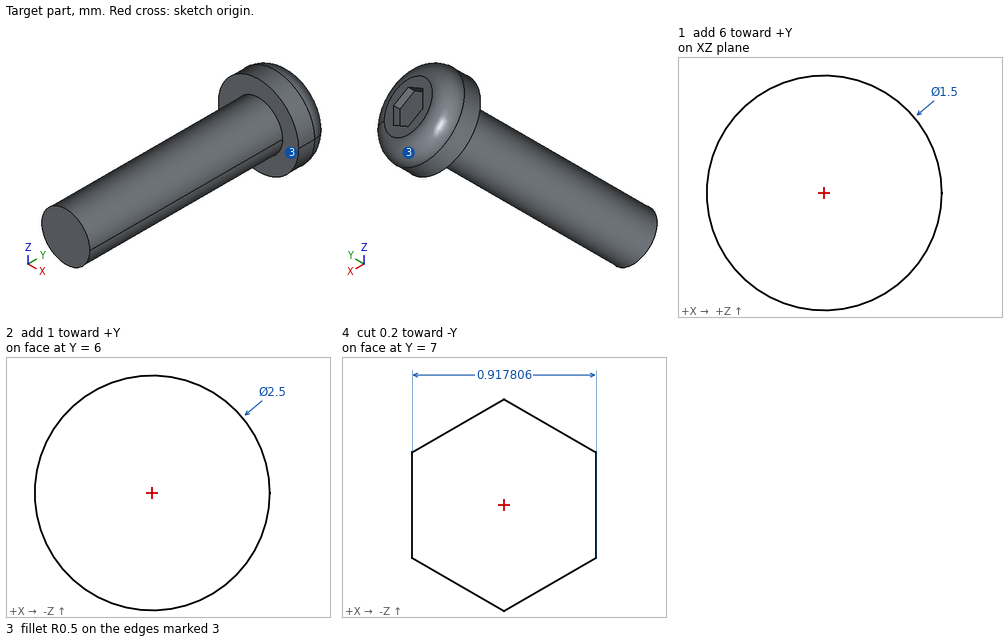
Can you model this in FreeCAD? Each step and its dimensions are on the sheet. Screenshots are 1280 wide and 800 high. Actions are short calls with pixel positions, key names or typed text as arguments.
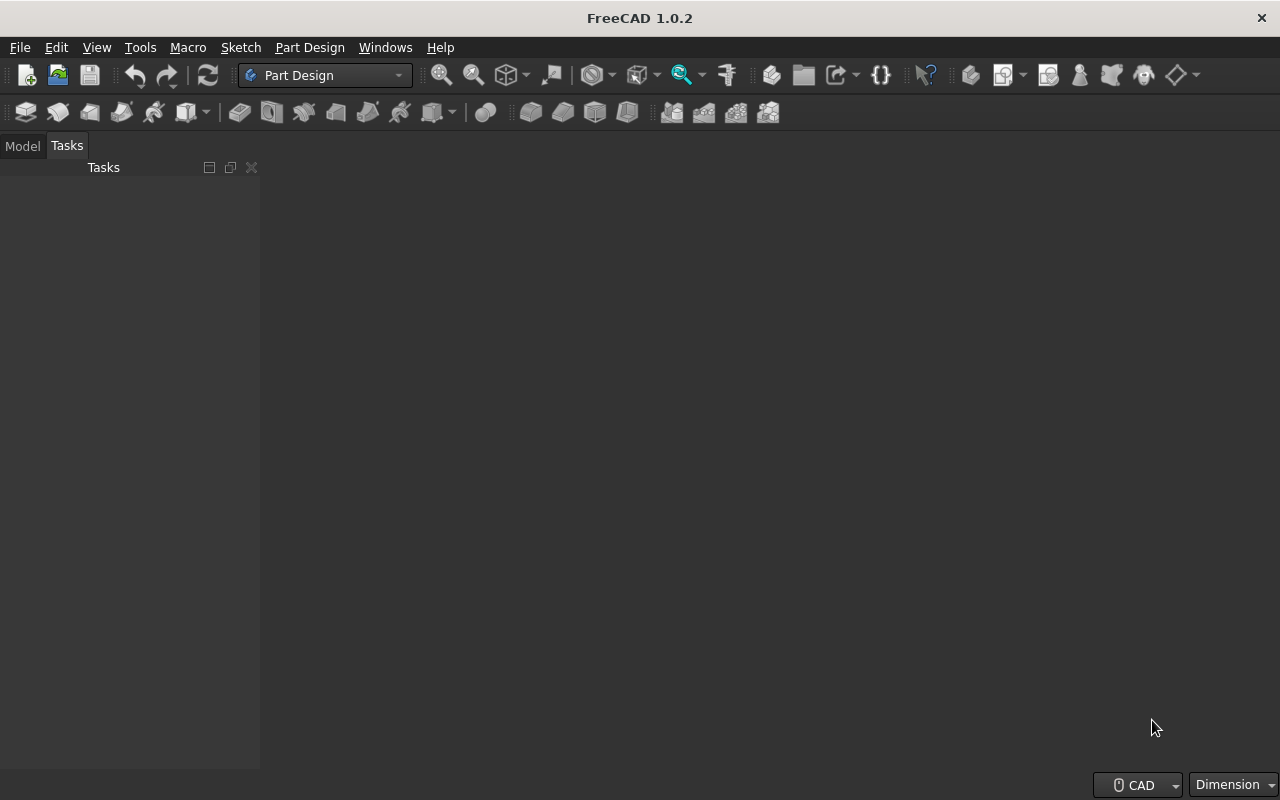
key(ctrl+n)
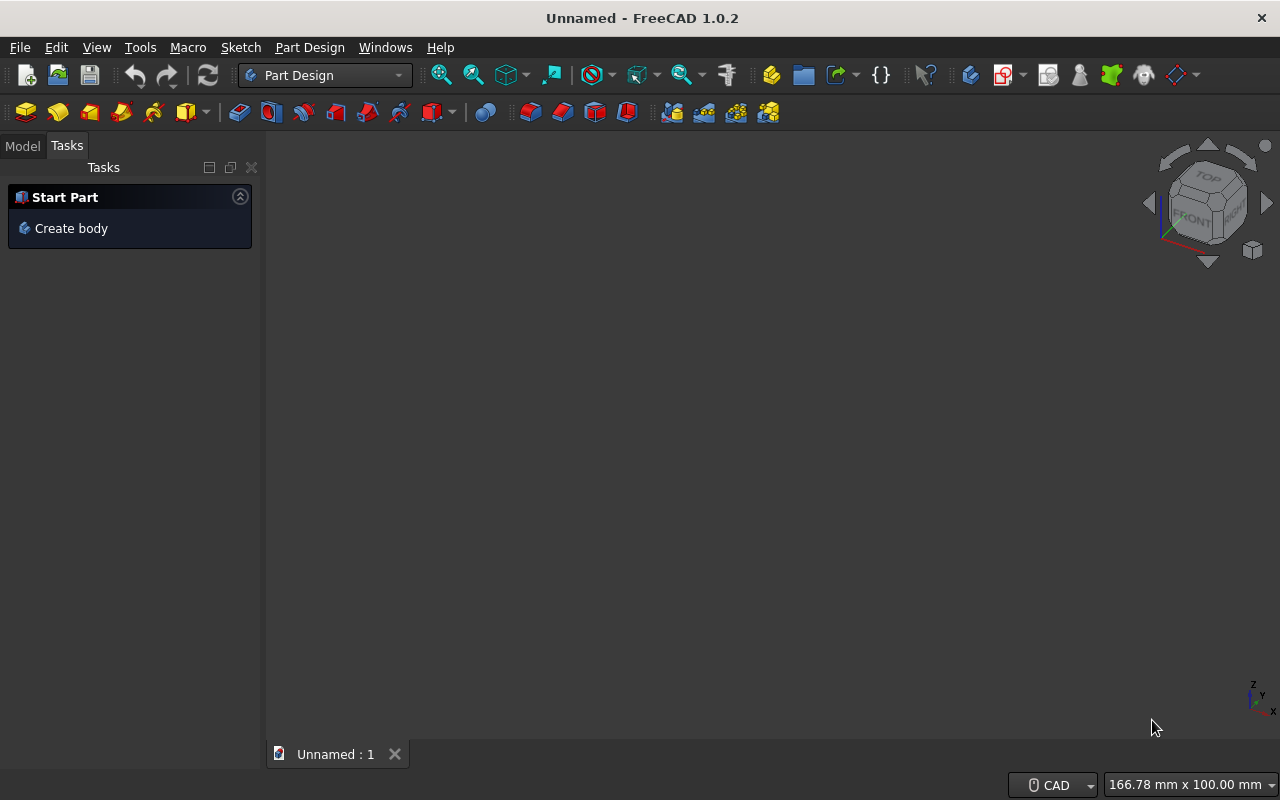
click(1004, 76)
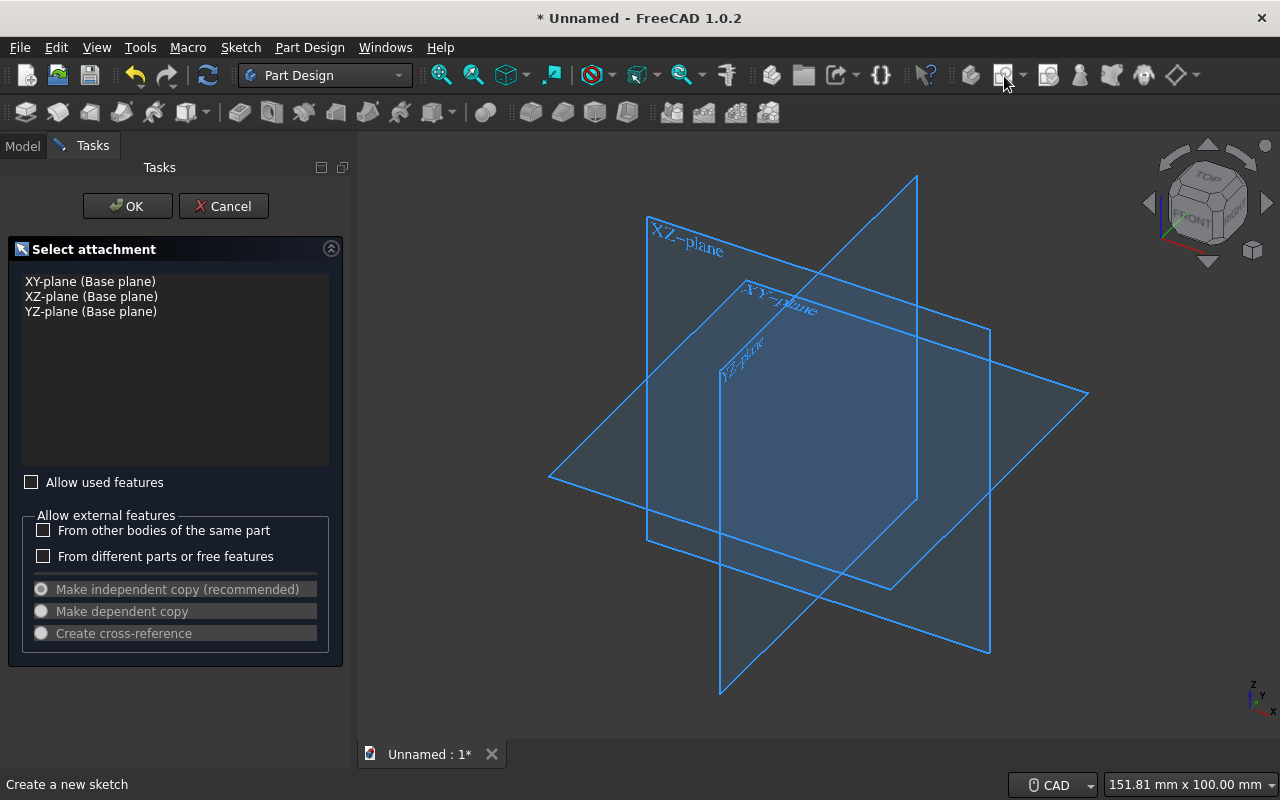
click(82, 296)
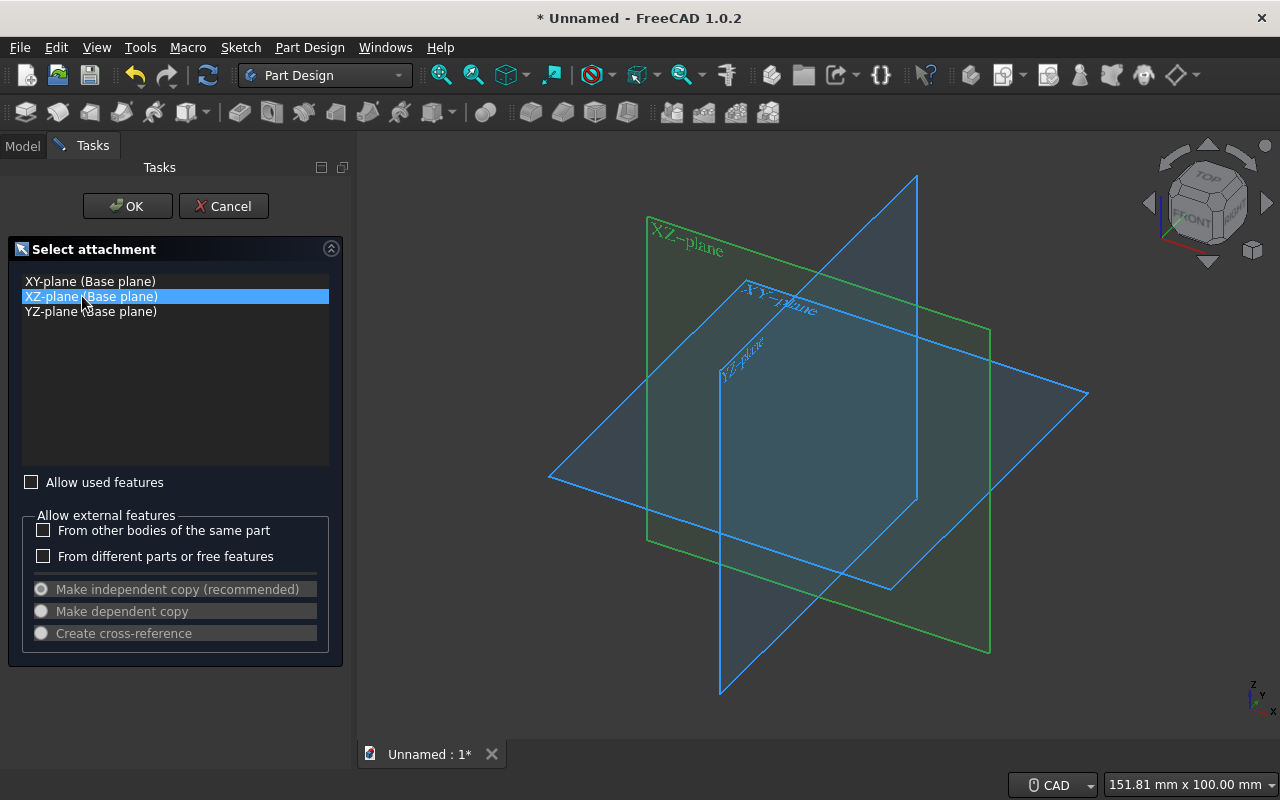
click(128, 206)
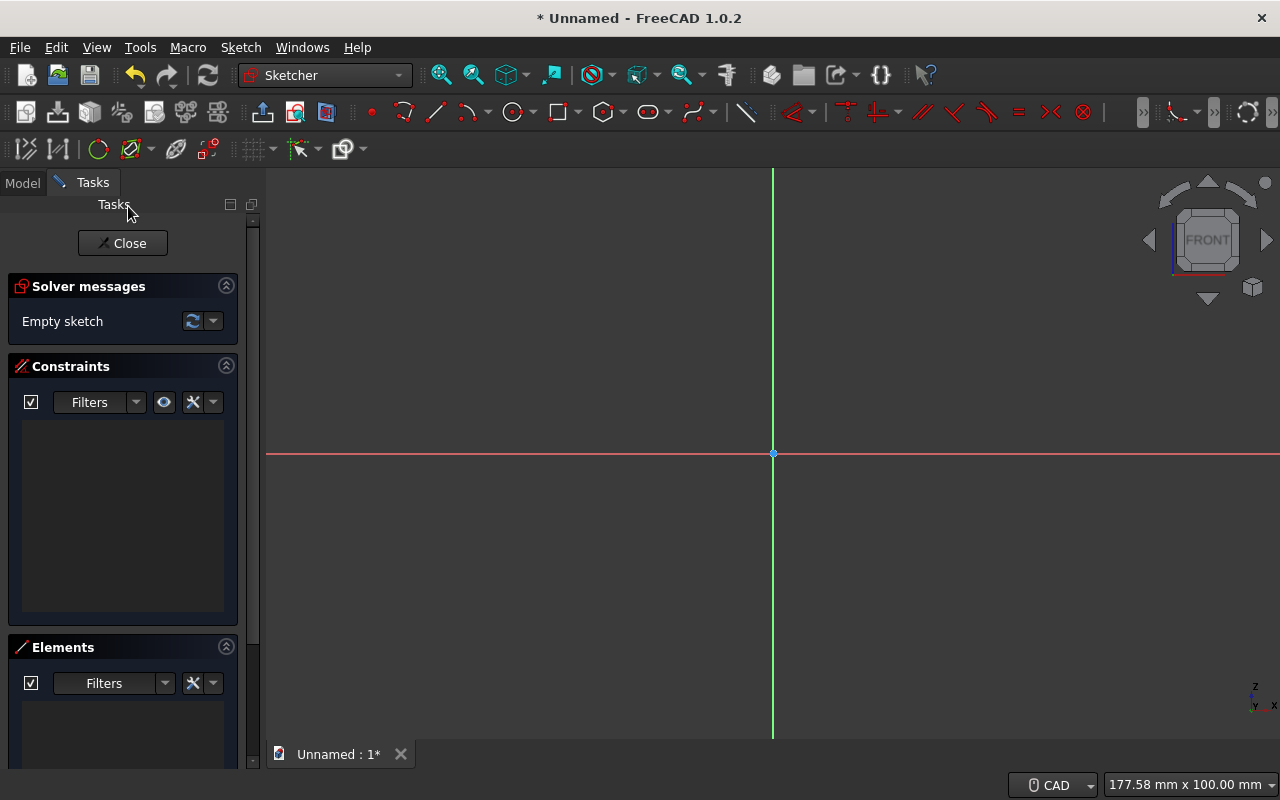
scroll(777, 454, up, 15)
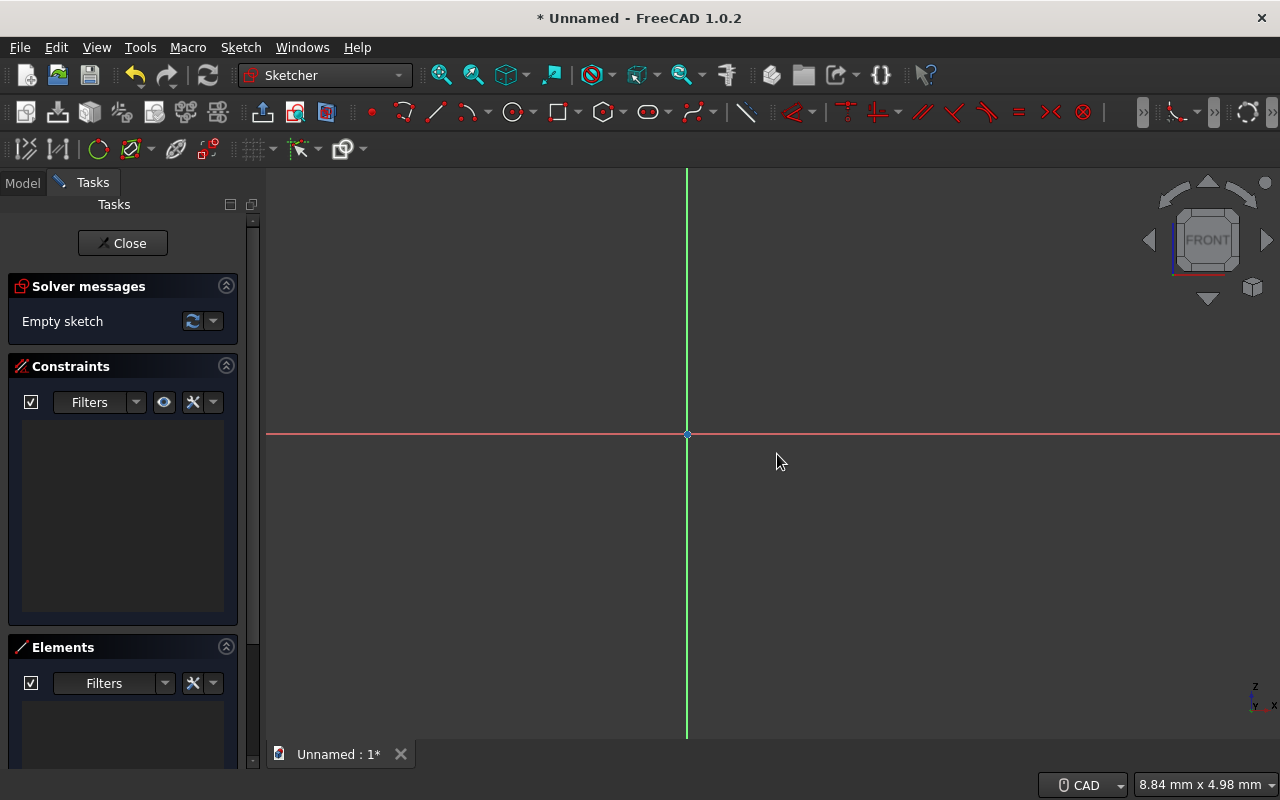
scroll(673, 419, up, 4)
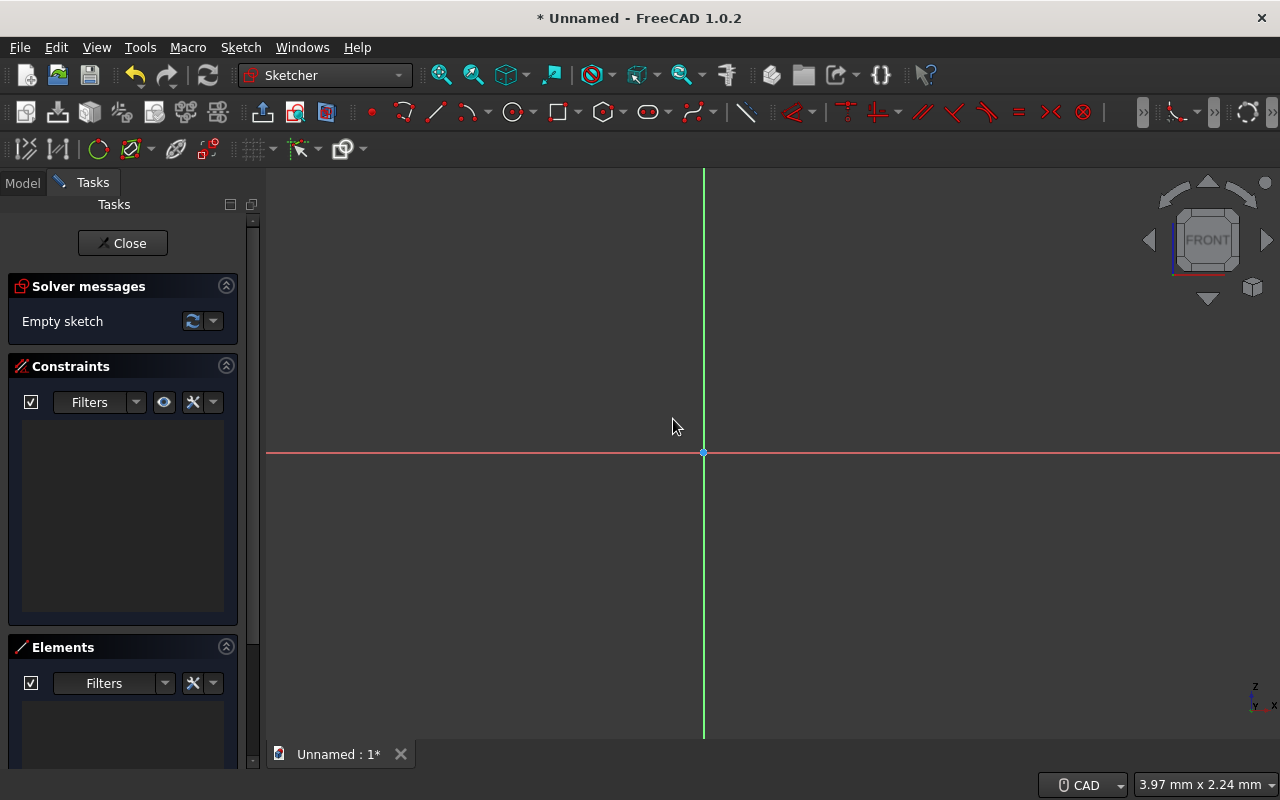
click(514, 112)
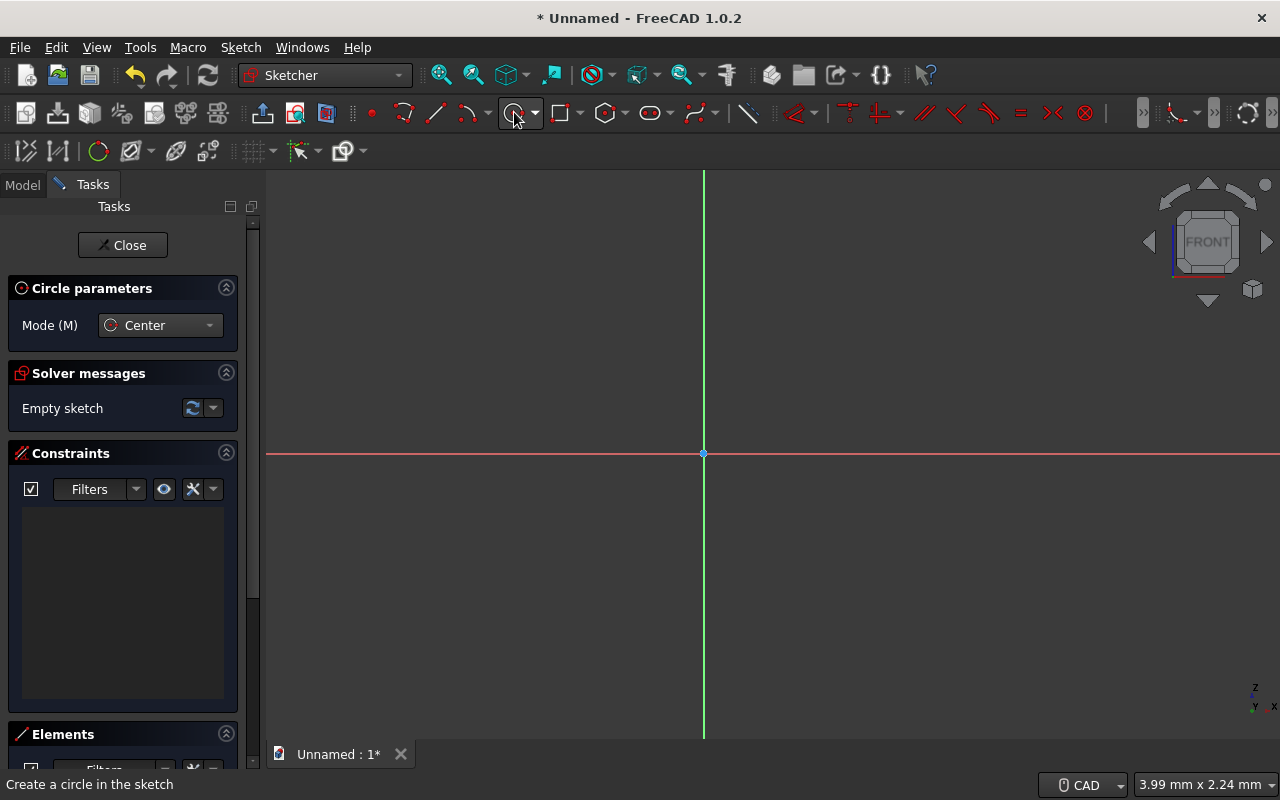
click(704, 454)
click(839, 319)
key(Escape)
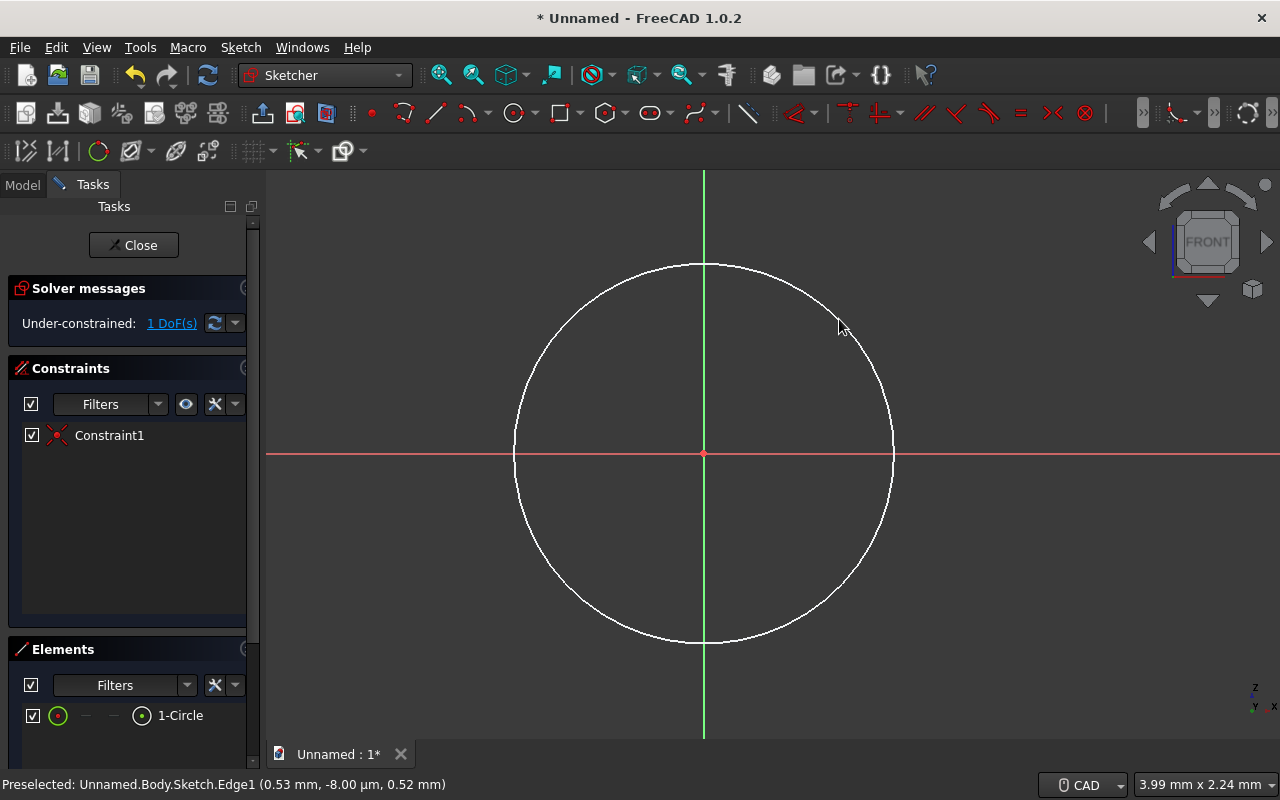
click(838, 319)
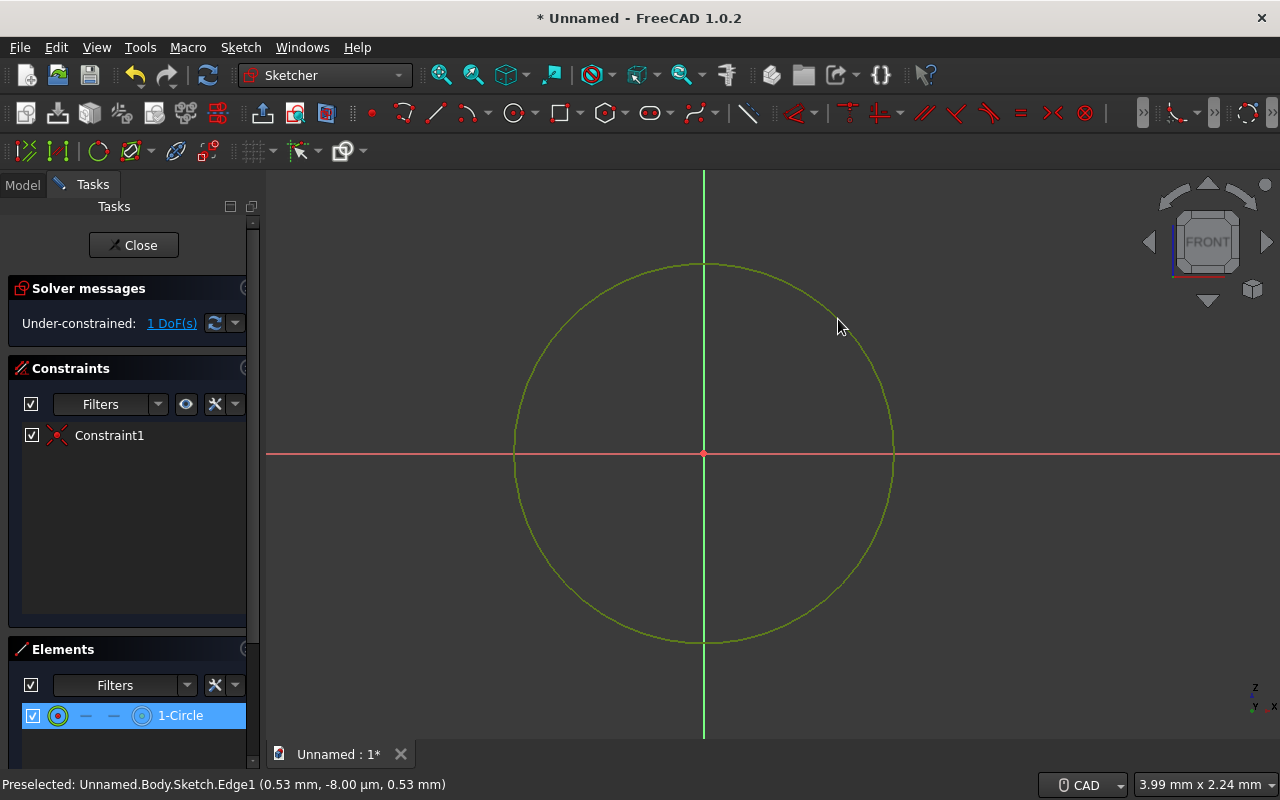
key(k)
key(o)